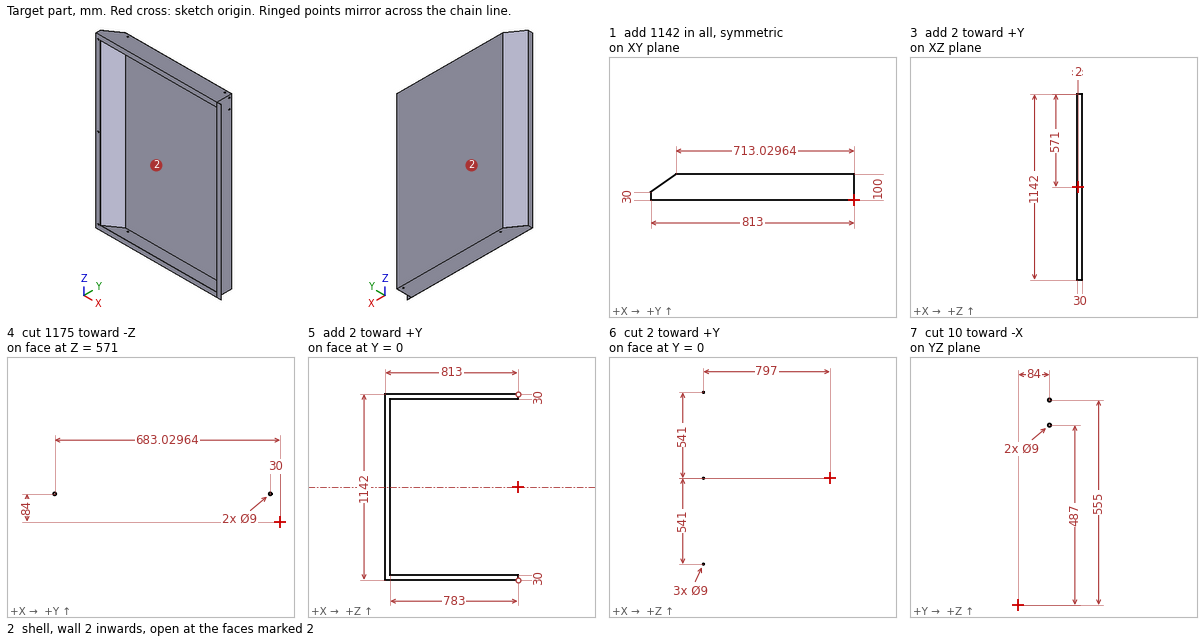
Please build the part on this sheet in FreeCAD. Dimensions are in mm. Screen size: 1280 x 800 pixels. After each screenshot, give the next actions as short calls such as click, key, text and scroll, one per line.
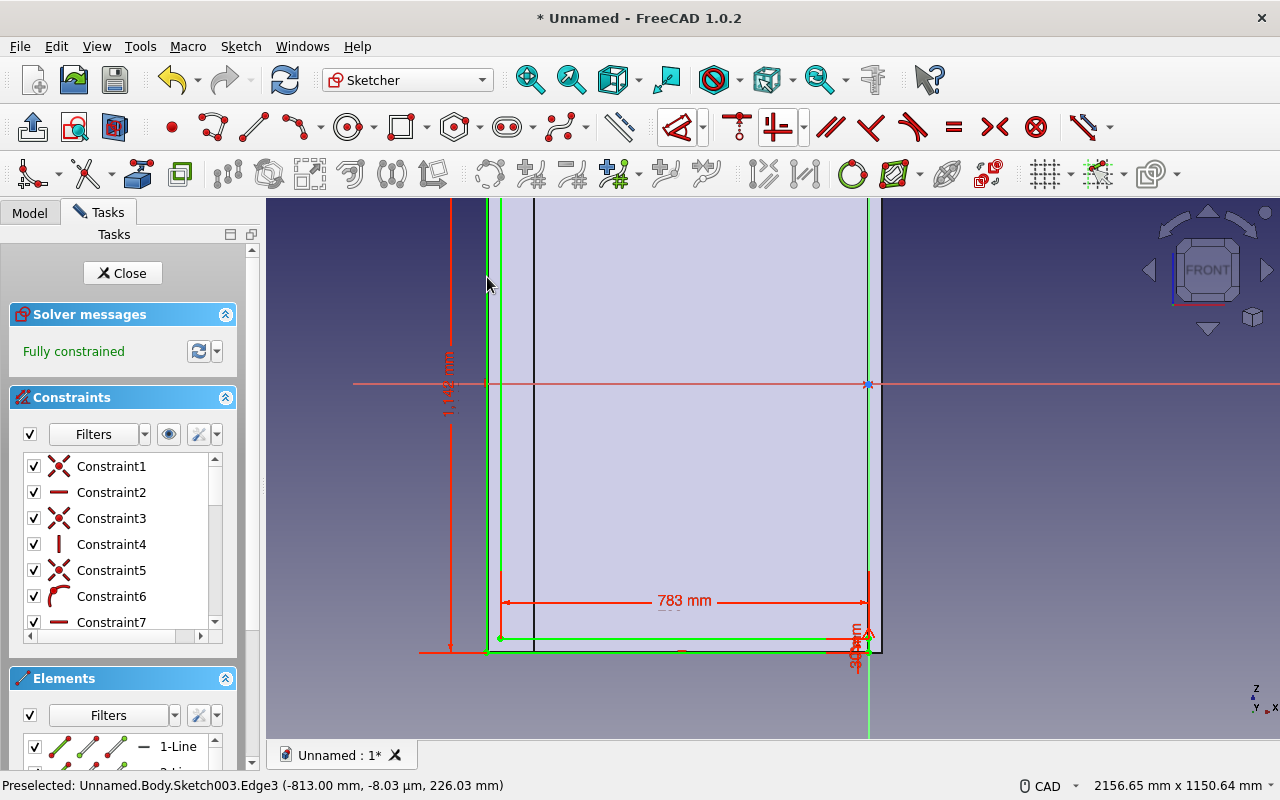
click(123, 273)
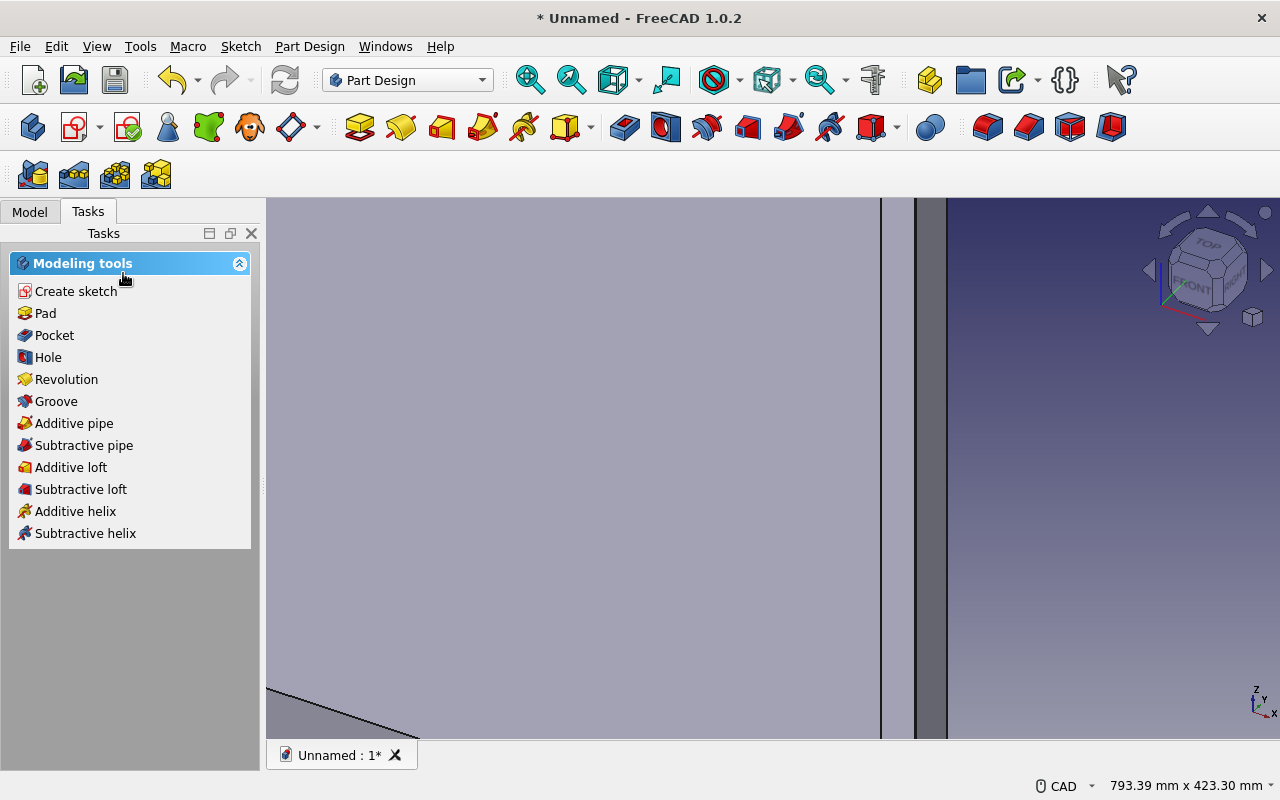
click(360, 128)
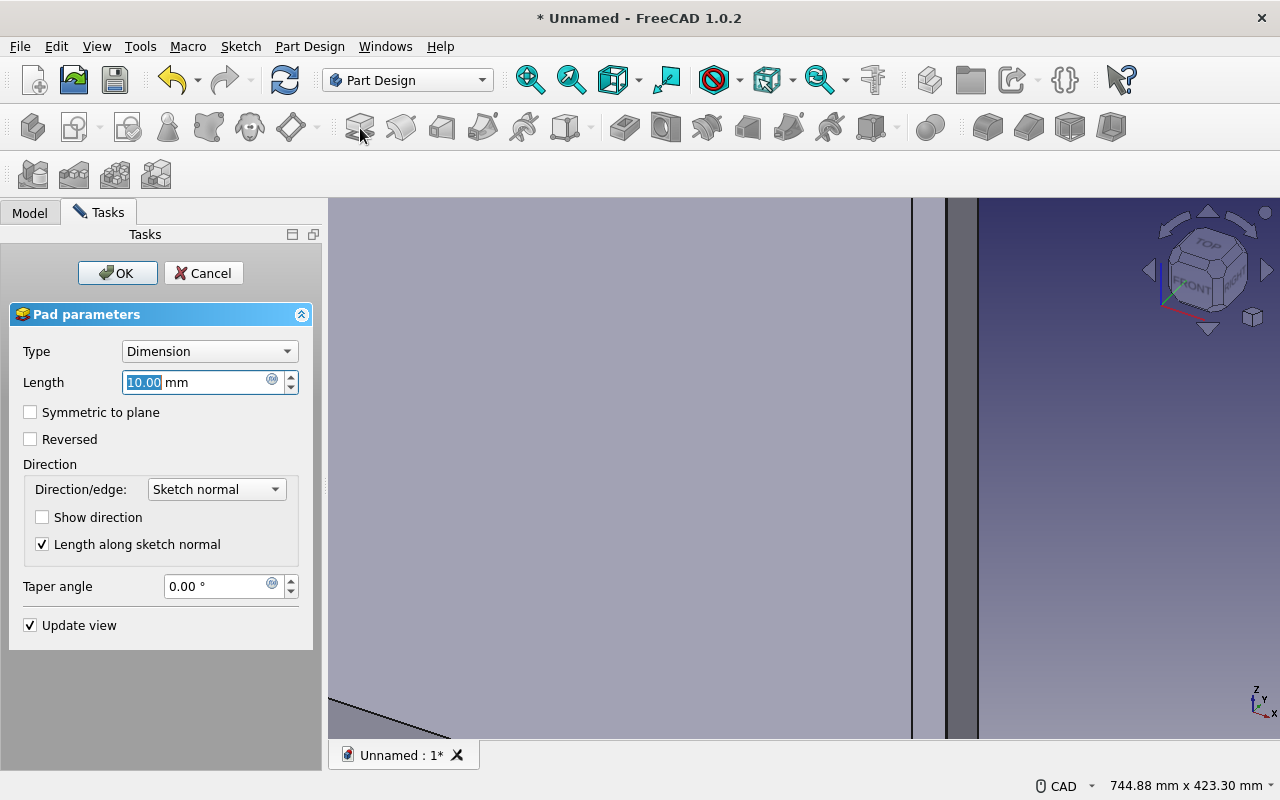
text(2)
key(Tab)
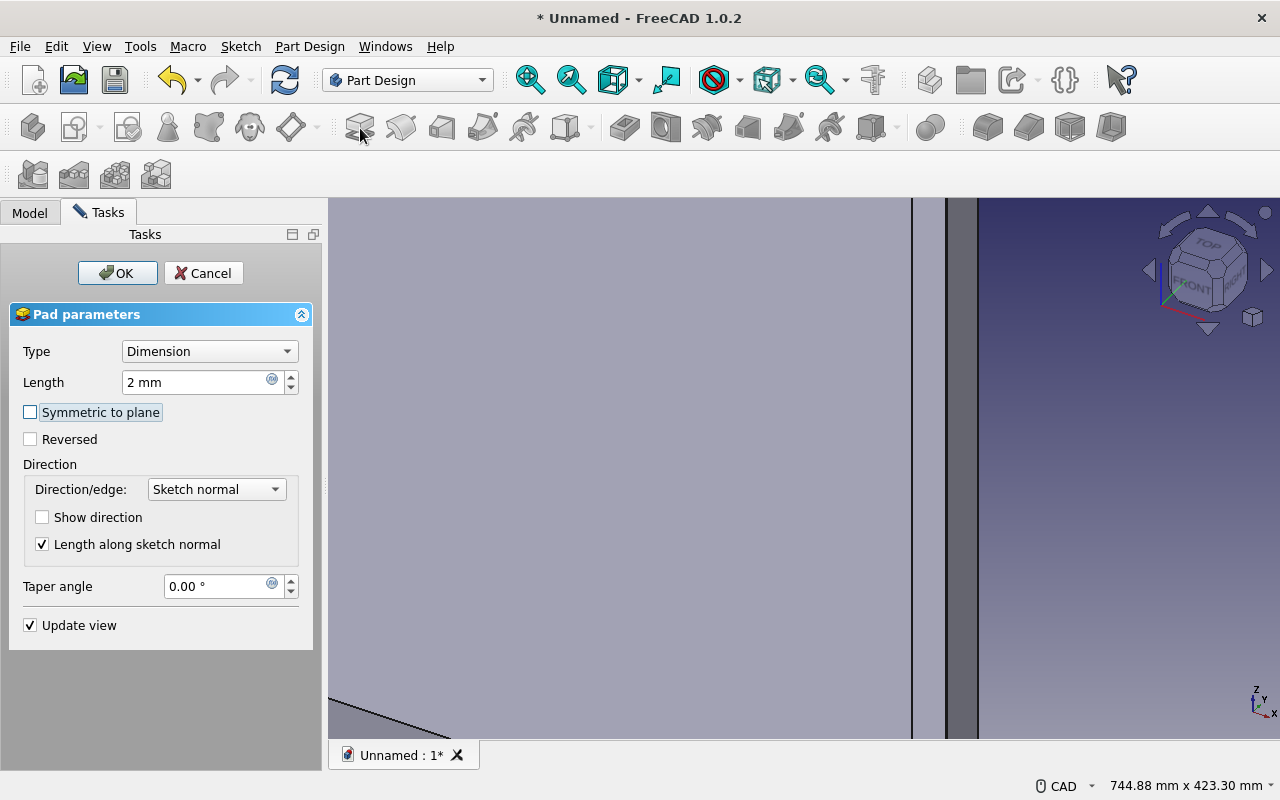
click(31, 439)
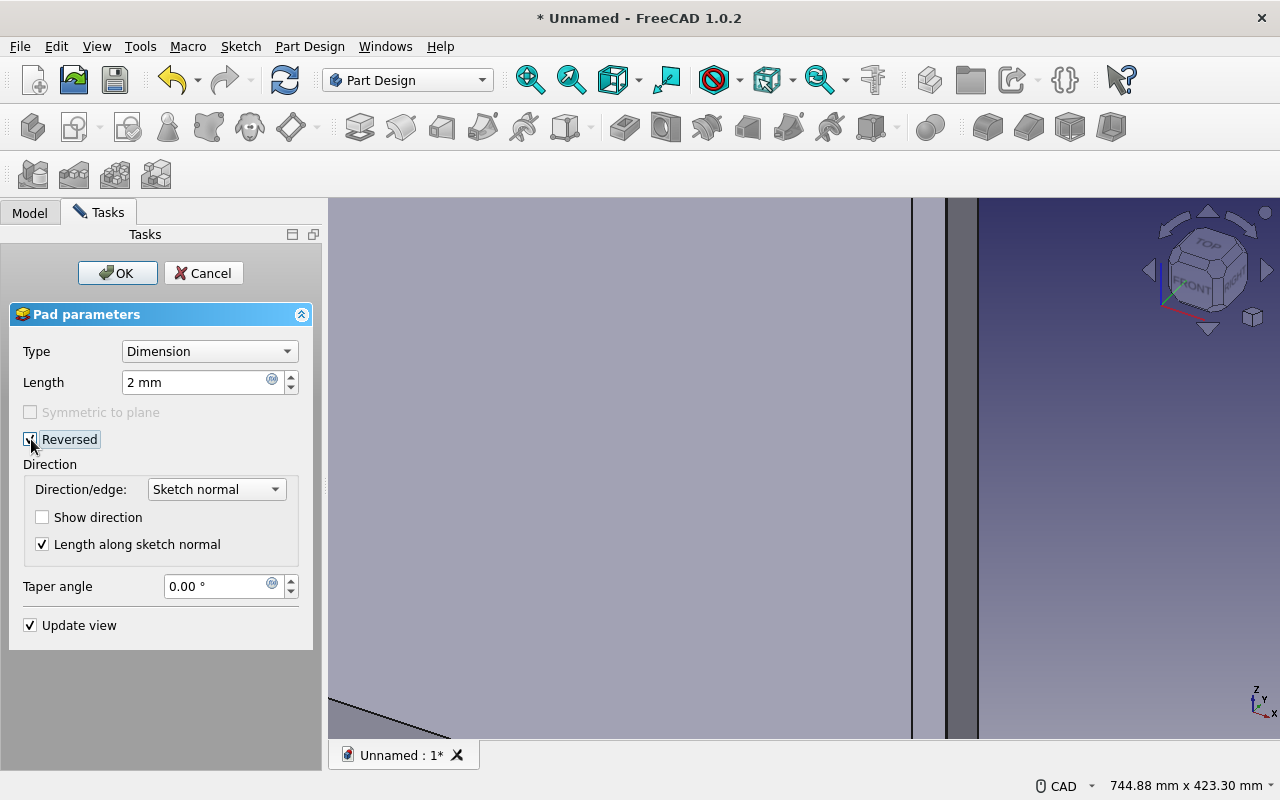
click(118, 273)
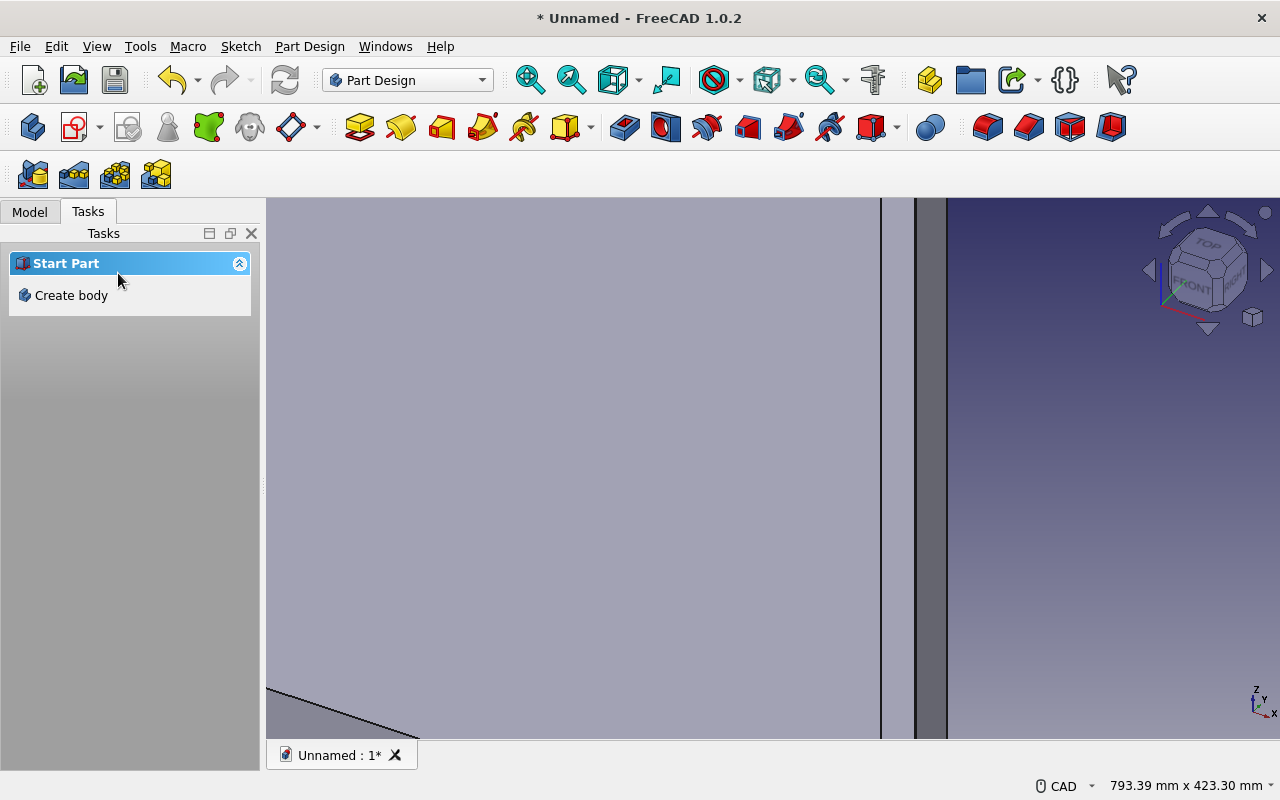
click(531, 80)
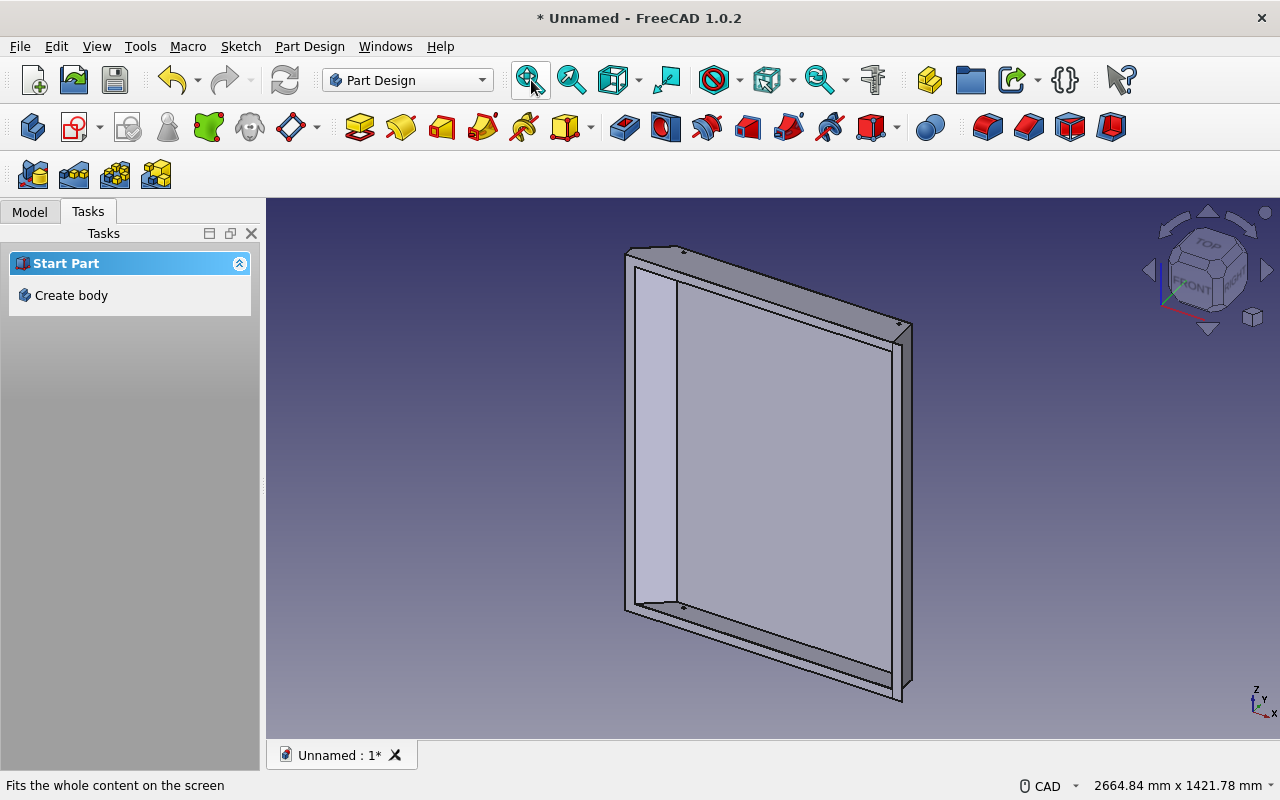
scroll(899, 466, up, 6)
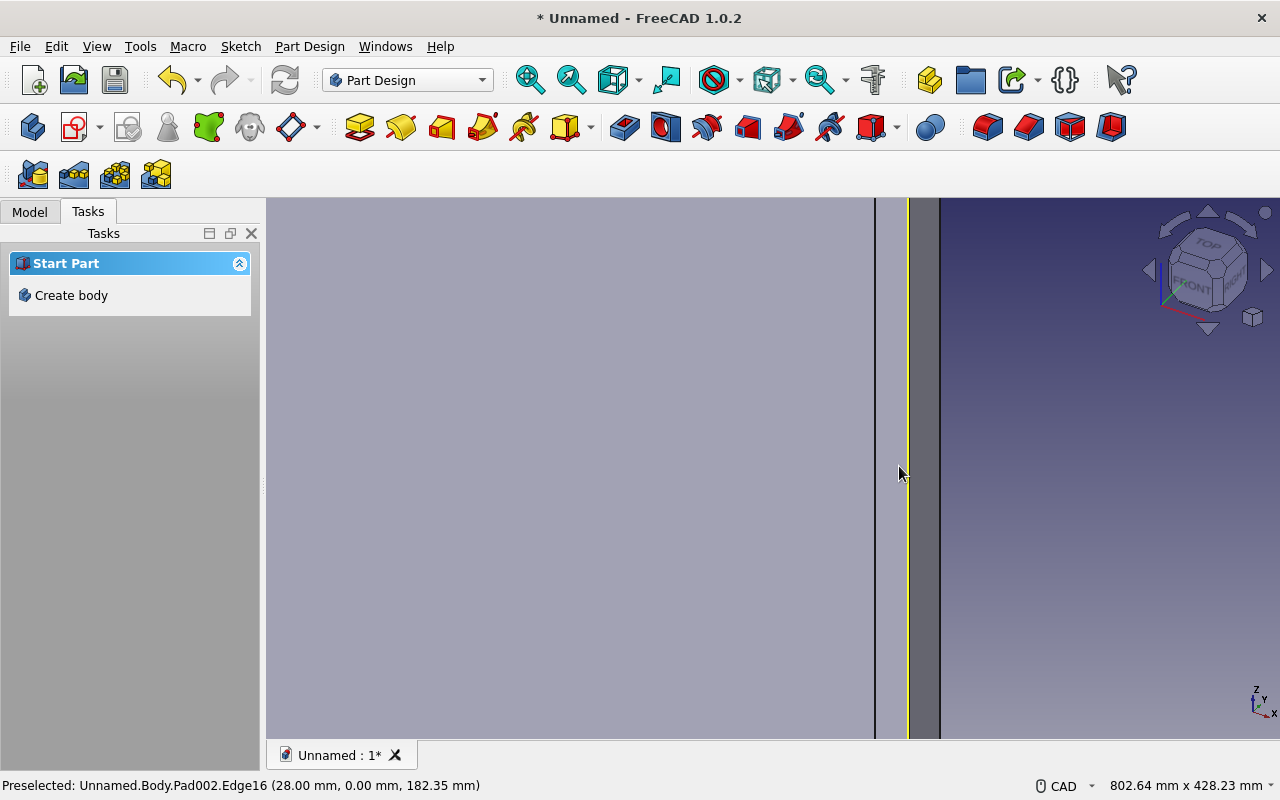
click(897, 466)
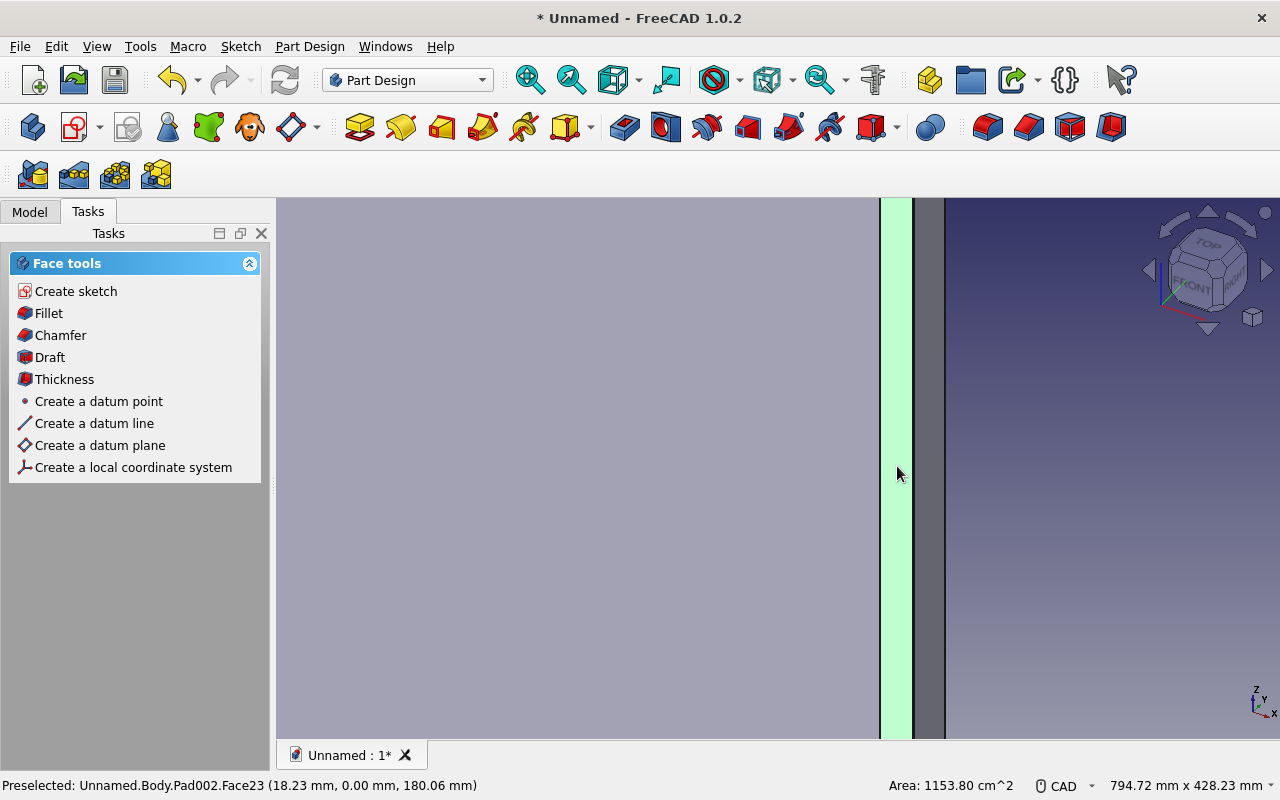
click(74, 128)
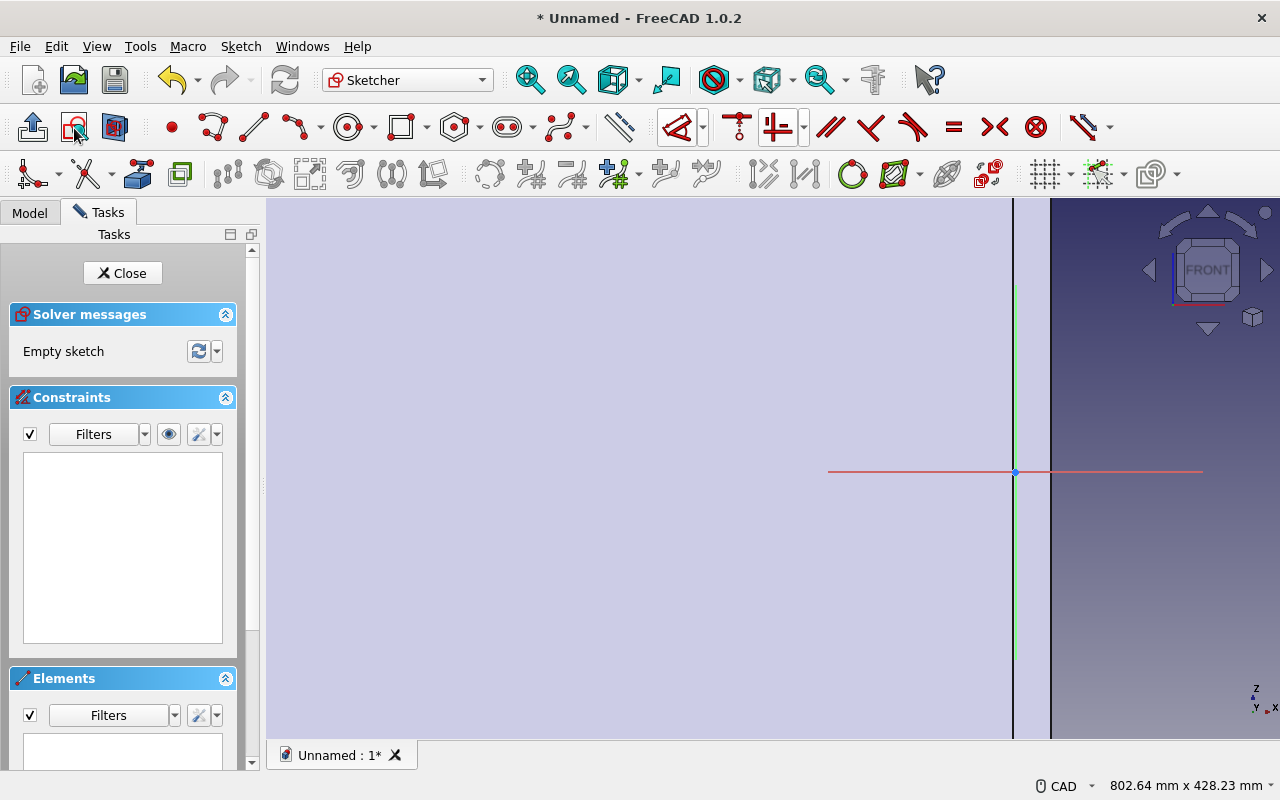
scroll(768, 467, down, 7)